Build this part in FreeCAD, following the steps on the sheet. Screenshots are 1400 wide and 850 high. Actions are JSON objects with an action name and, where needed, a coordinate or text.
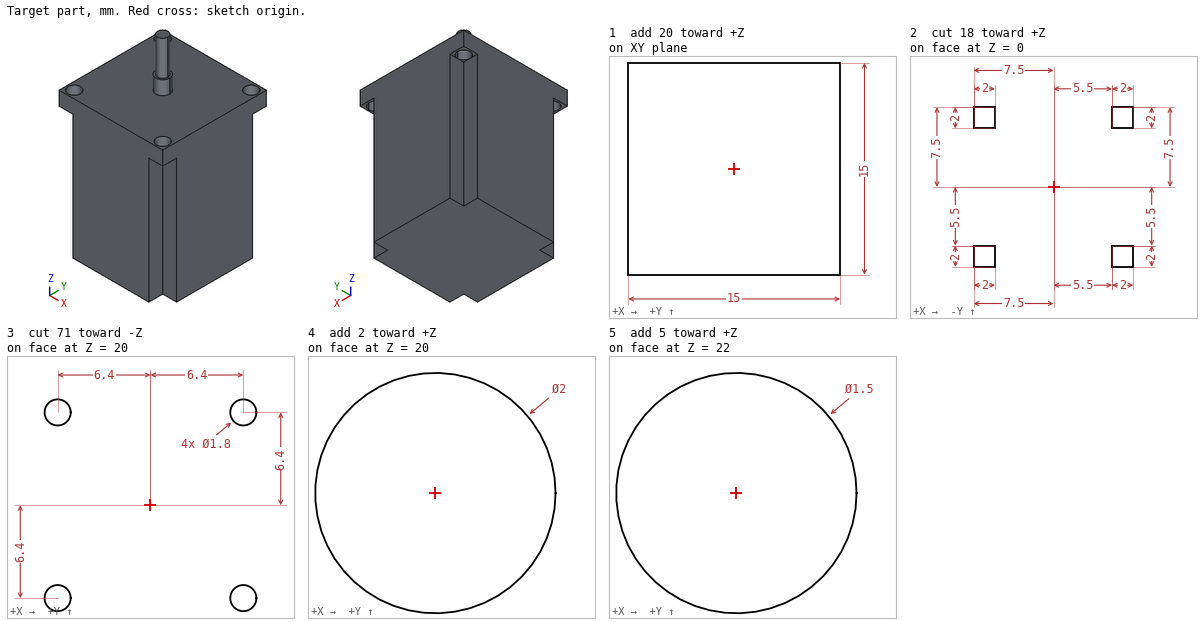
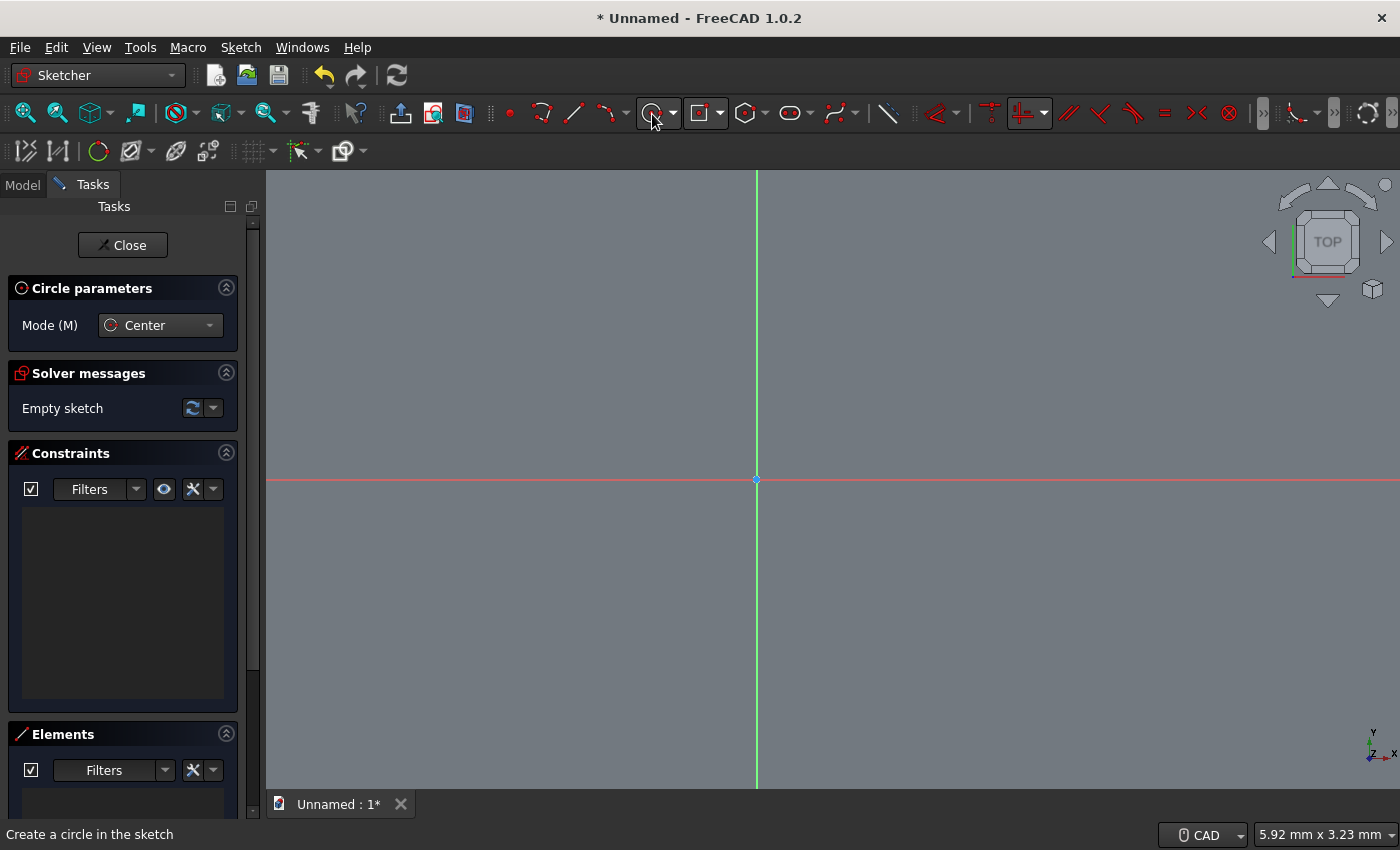
{"action": "left_click", "coordinate": [757, 479]}
{"action": "mouse_move", "coordinate": [892, 344]}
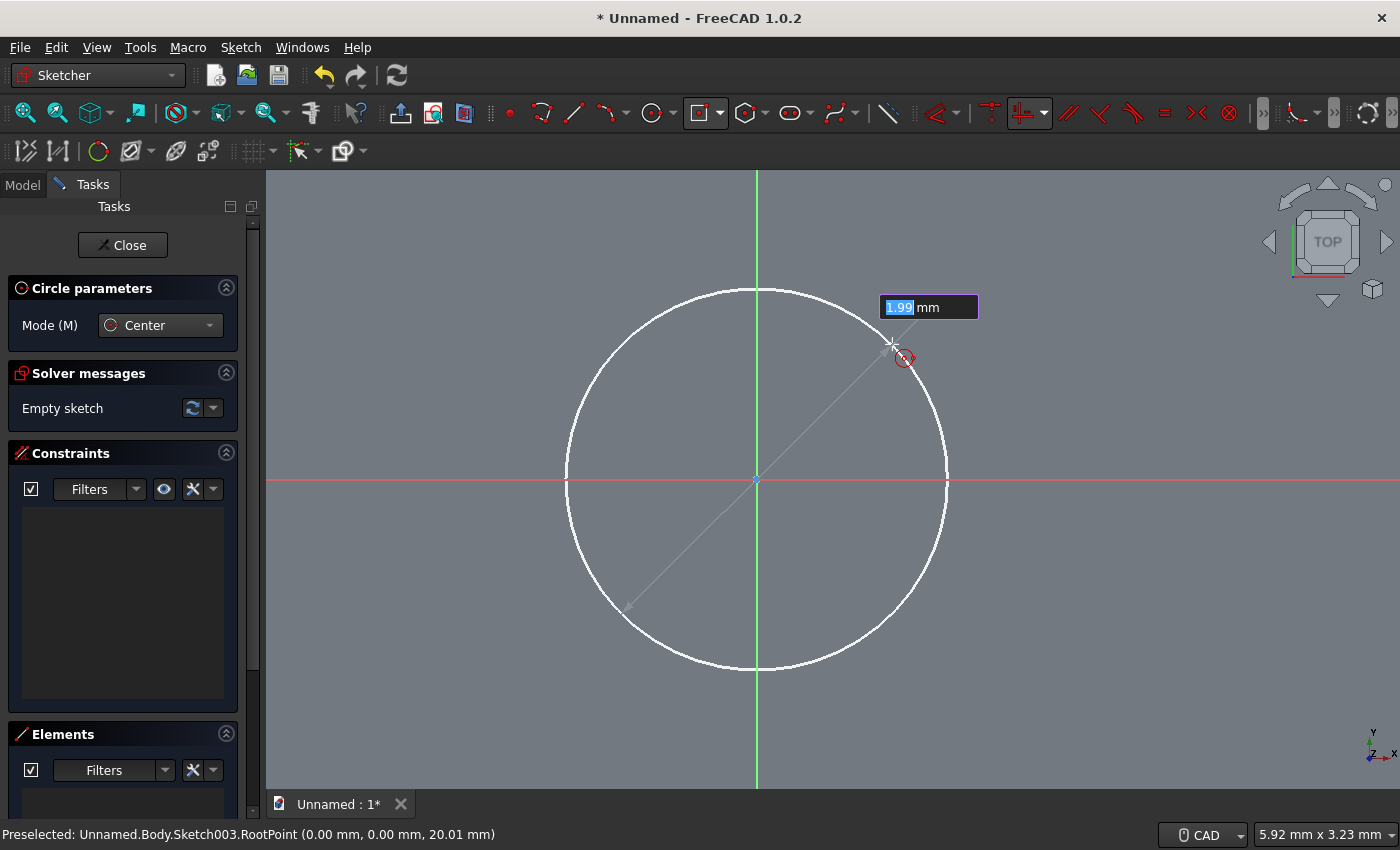
{"action": "type", "text": "2"}
{"action": "key", "text": "Return"}
{"action": "key", "text": "Escape"}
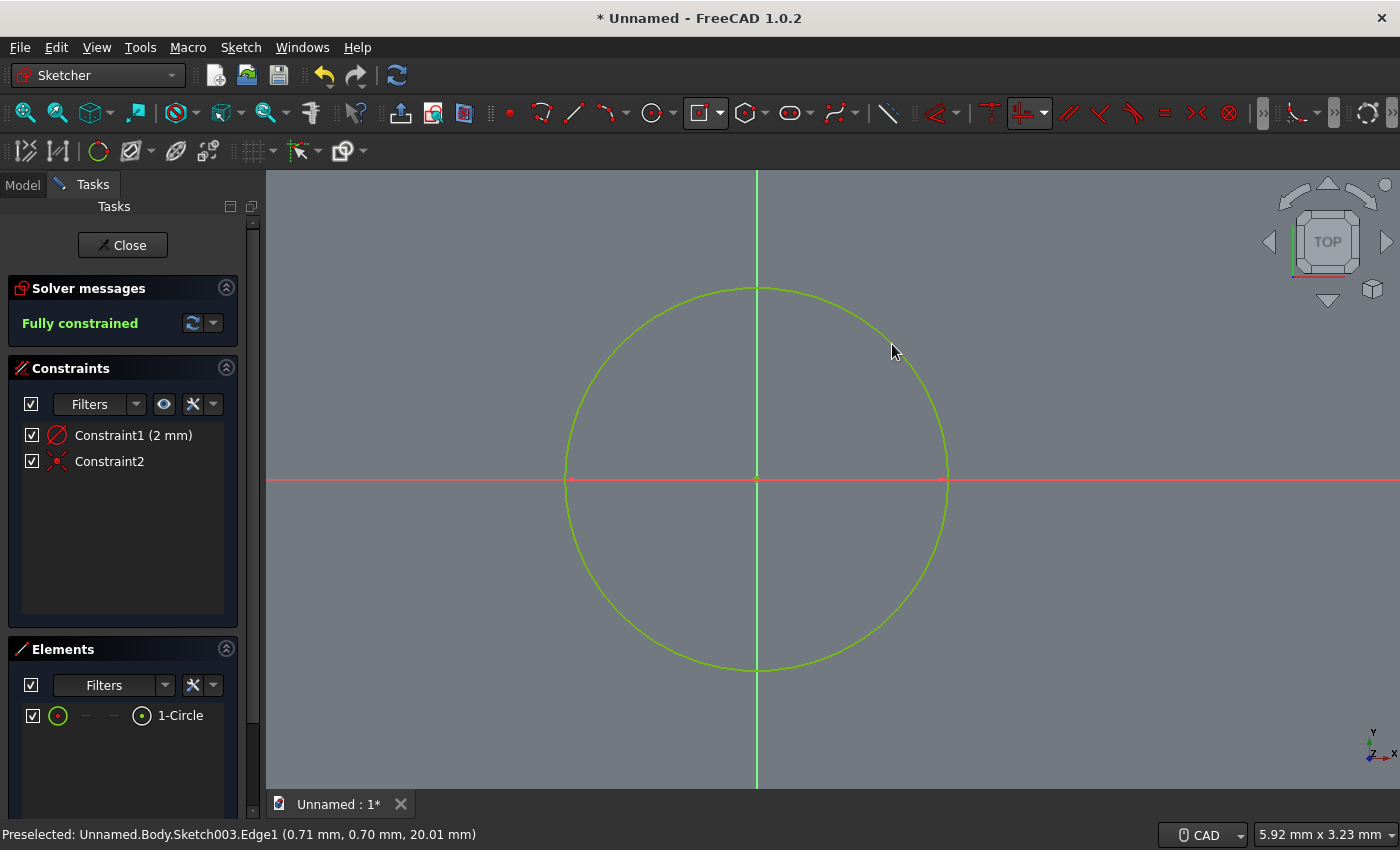
{"action": "left_click", "coordinate": [123, 245]}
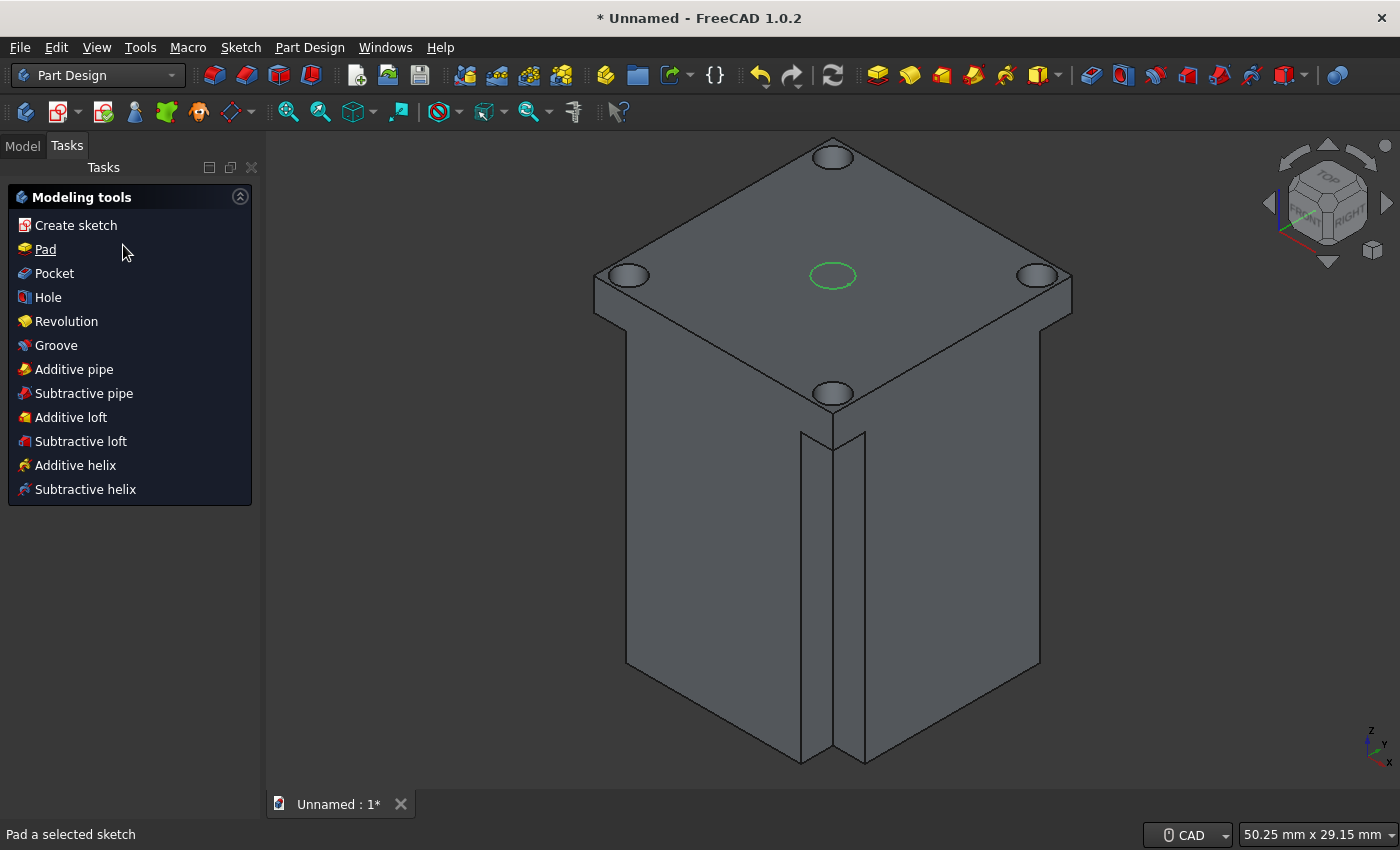
{"action": "left_click", "coordinate": [878, 76]}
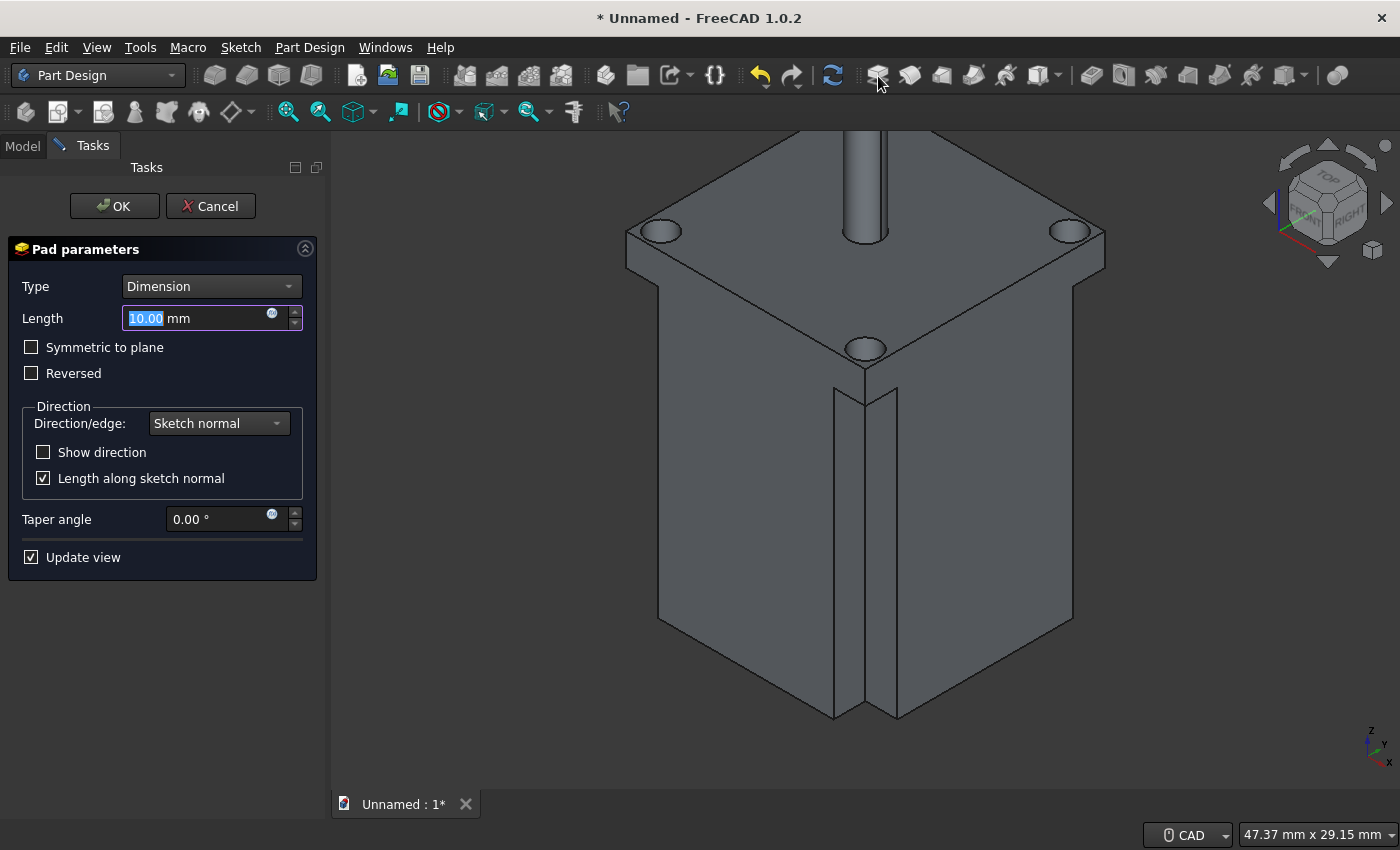
{"action": "type", "text": "2"}
{"action": "key", "text": "Tab"}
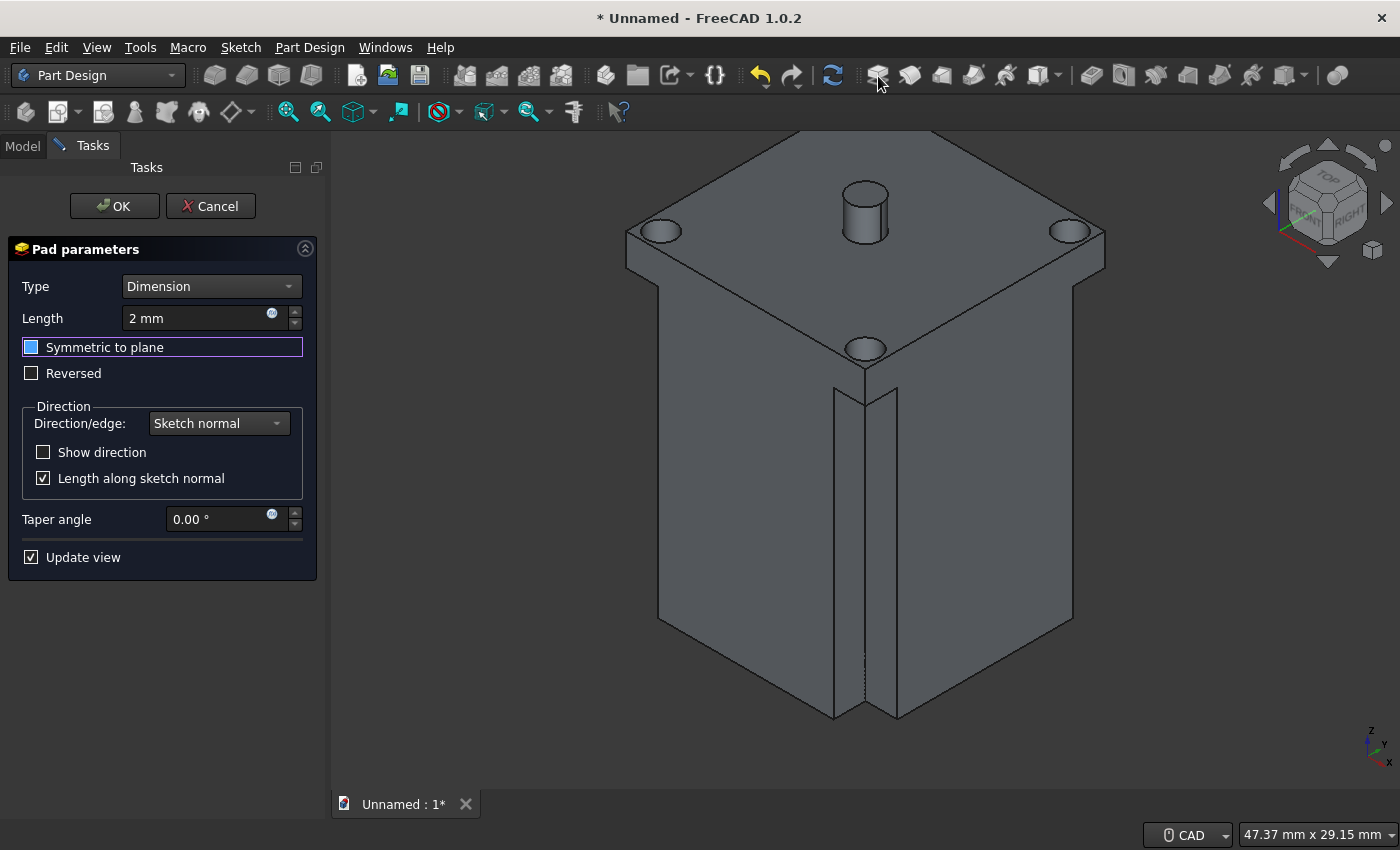
{"action": "left_click", "coordinate": [115, 206]}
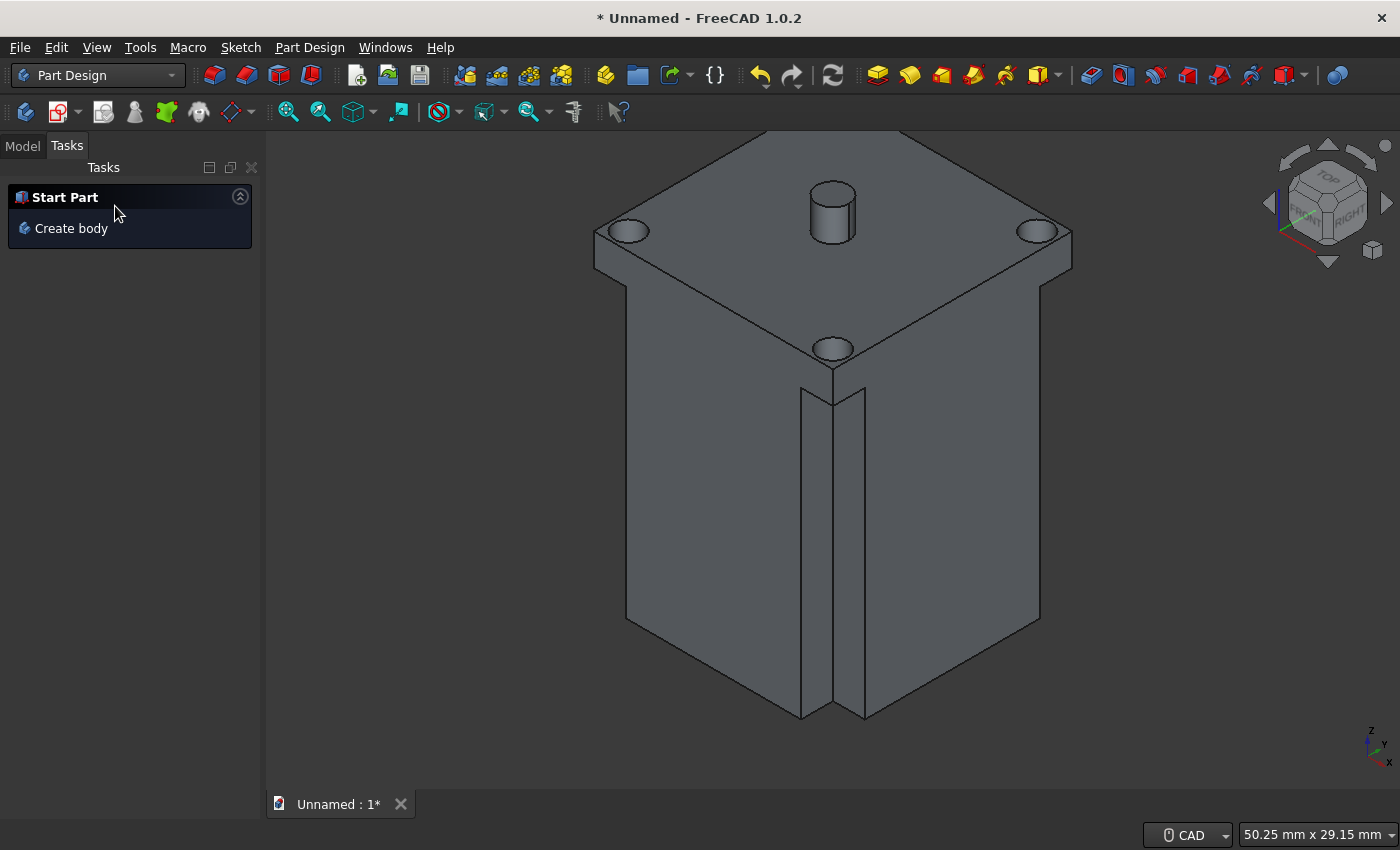
{"action": "left_click", "coordinate": [290, 112]}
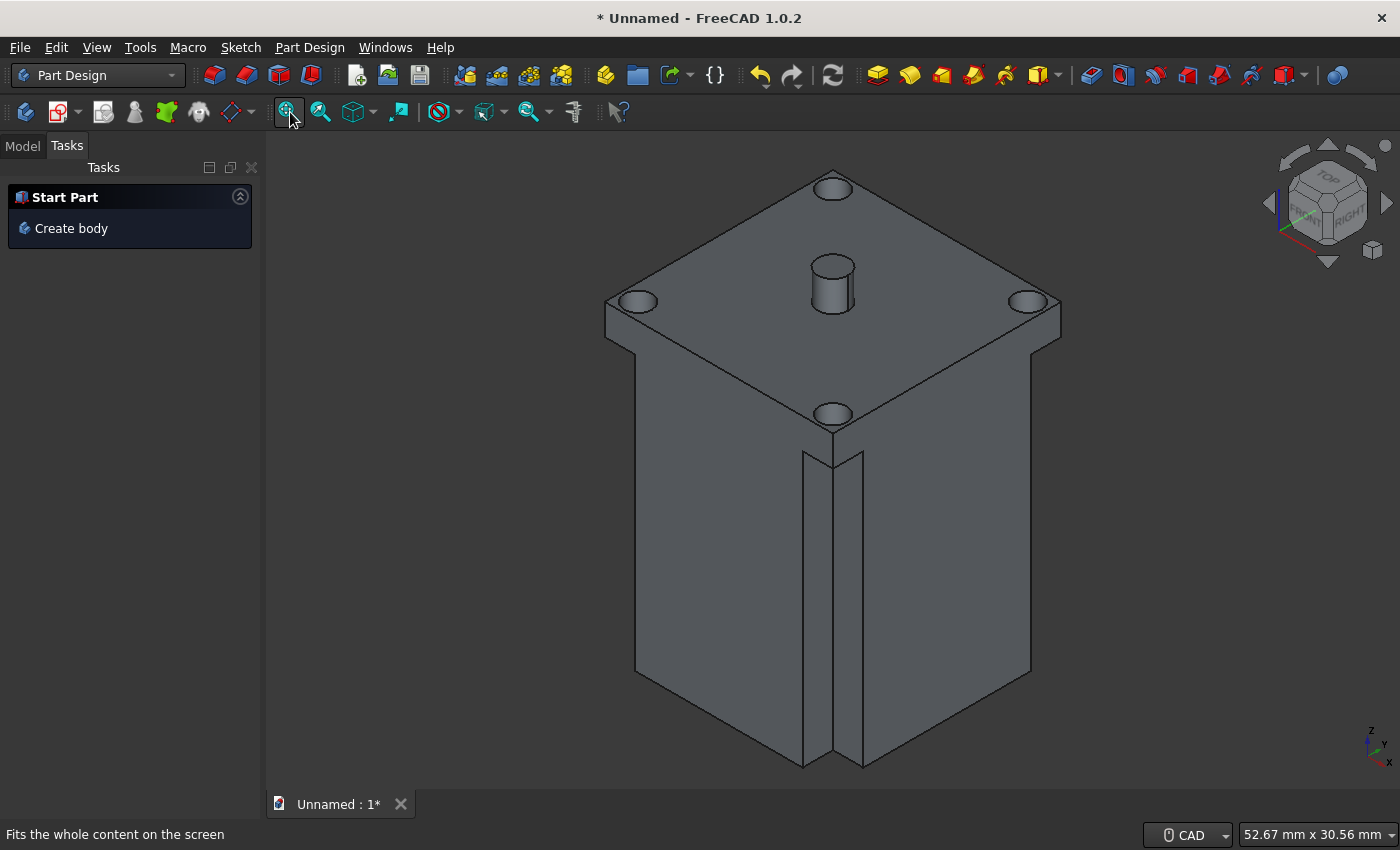
{"action": "left_click", "coordinate": [833, 266]}